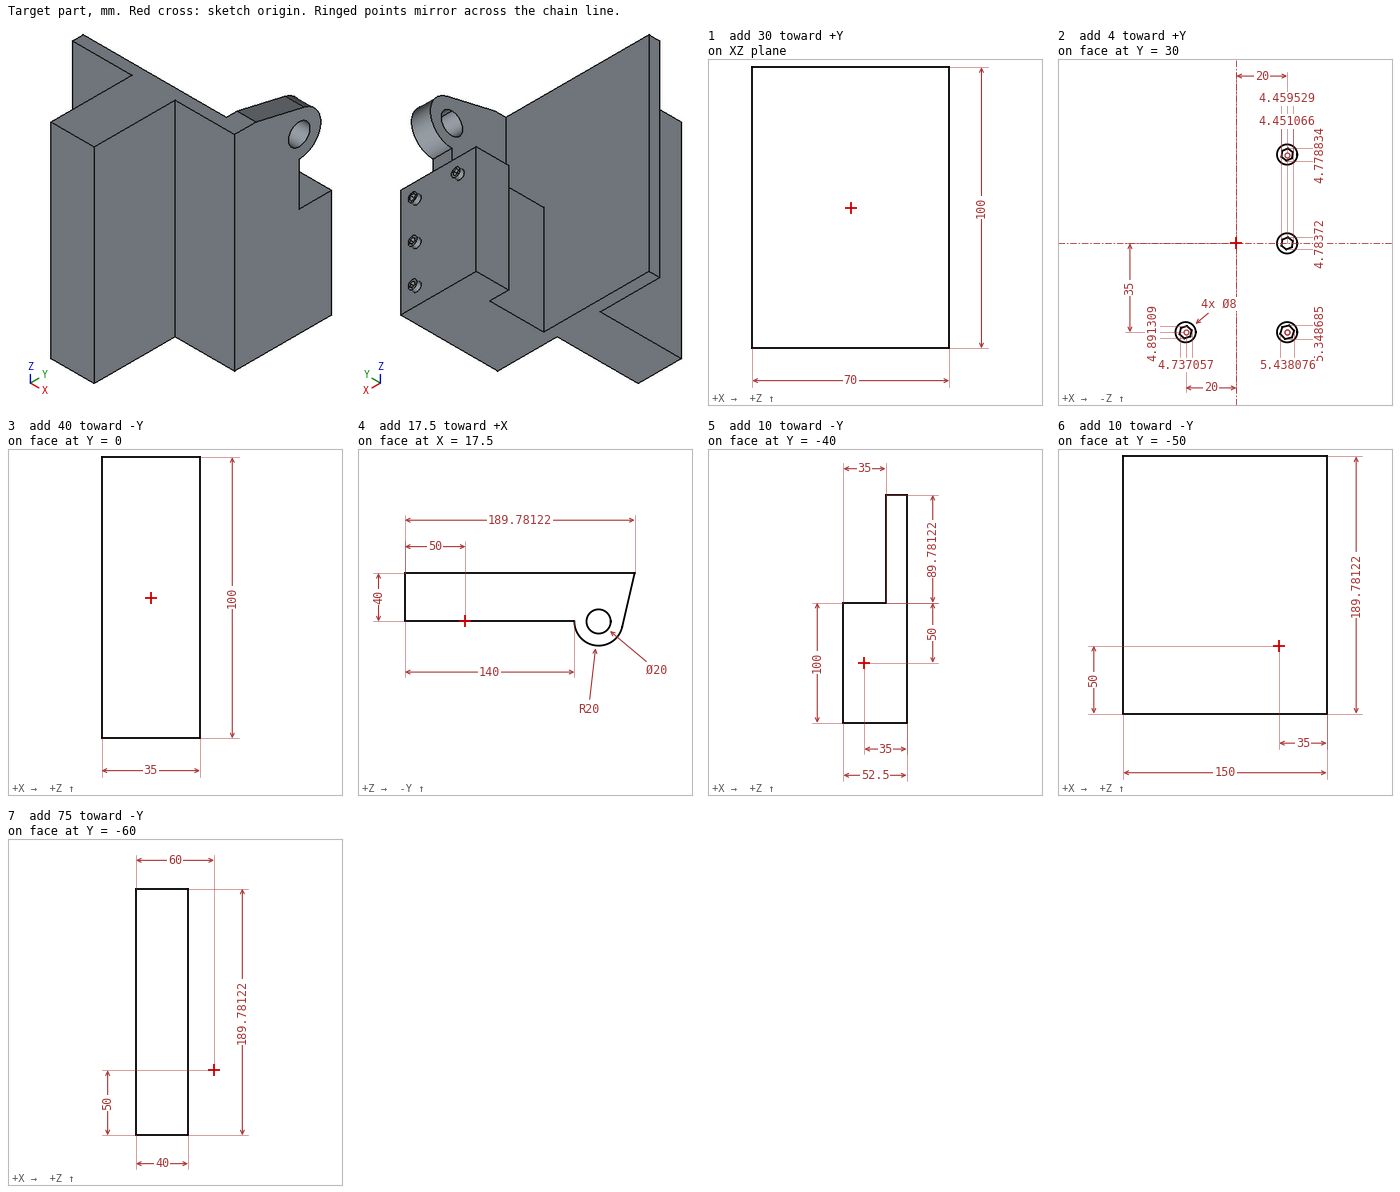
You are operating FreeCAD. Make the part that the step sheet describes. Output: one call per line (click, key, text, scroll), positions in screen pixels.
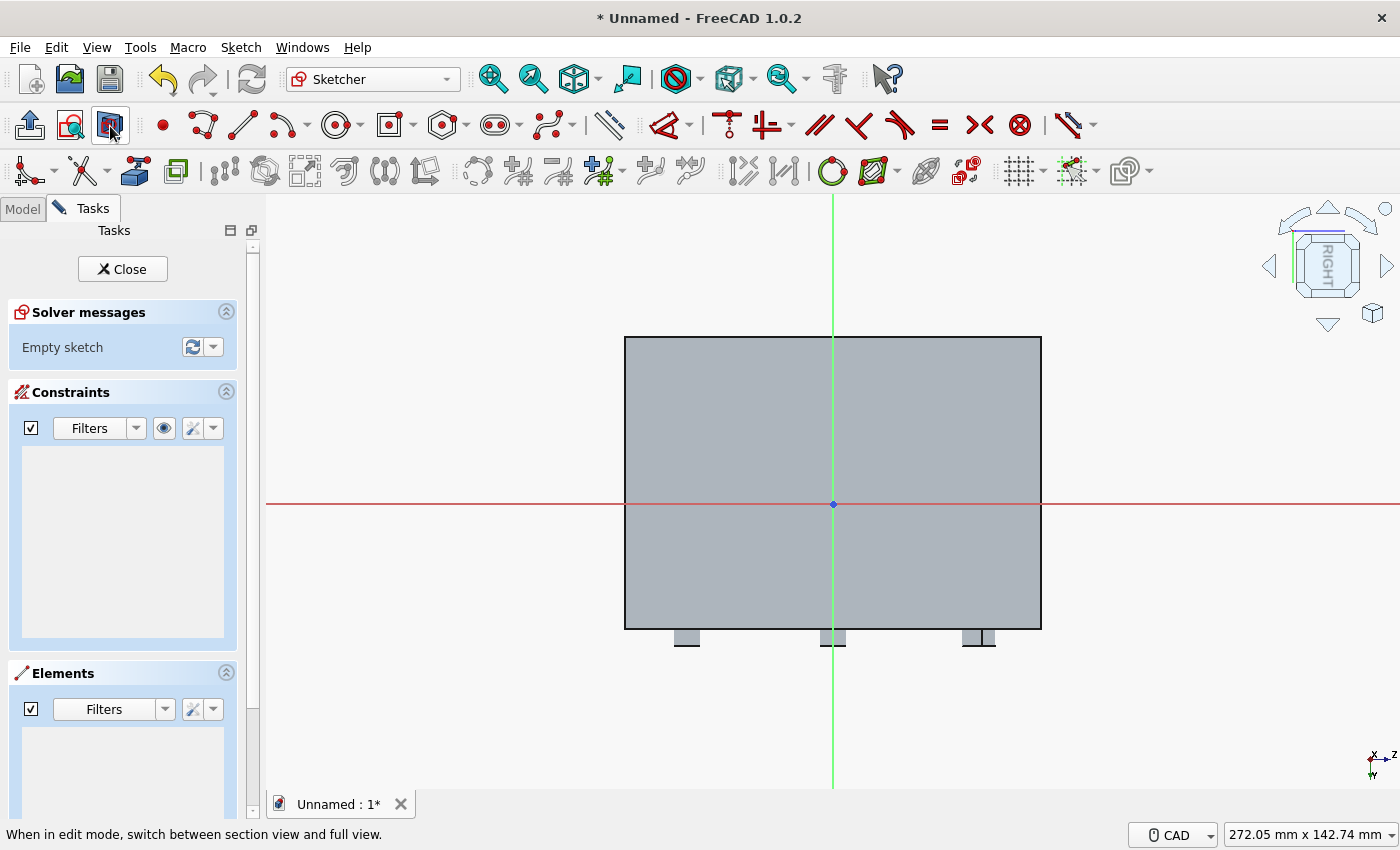
scroll(294, 551, down, 2)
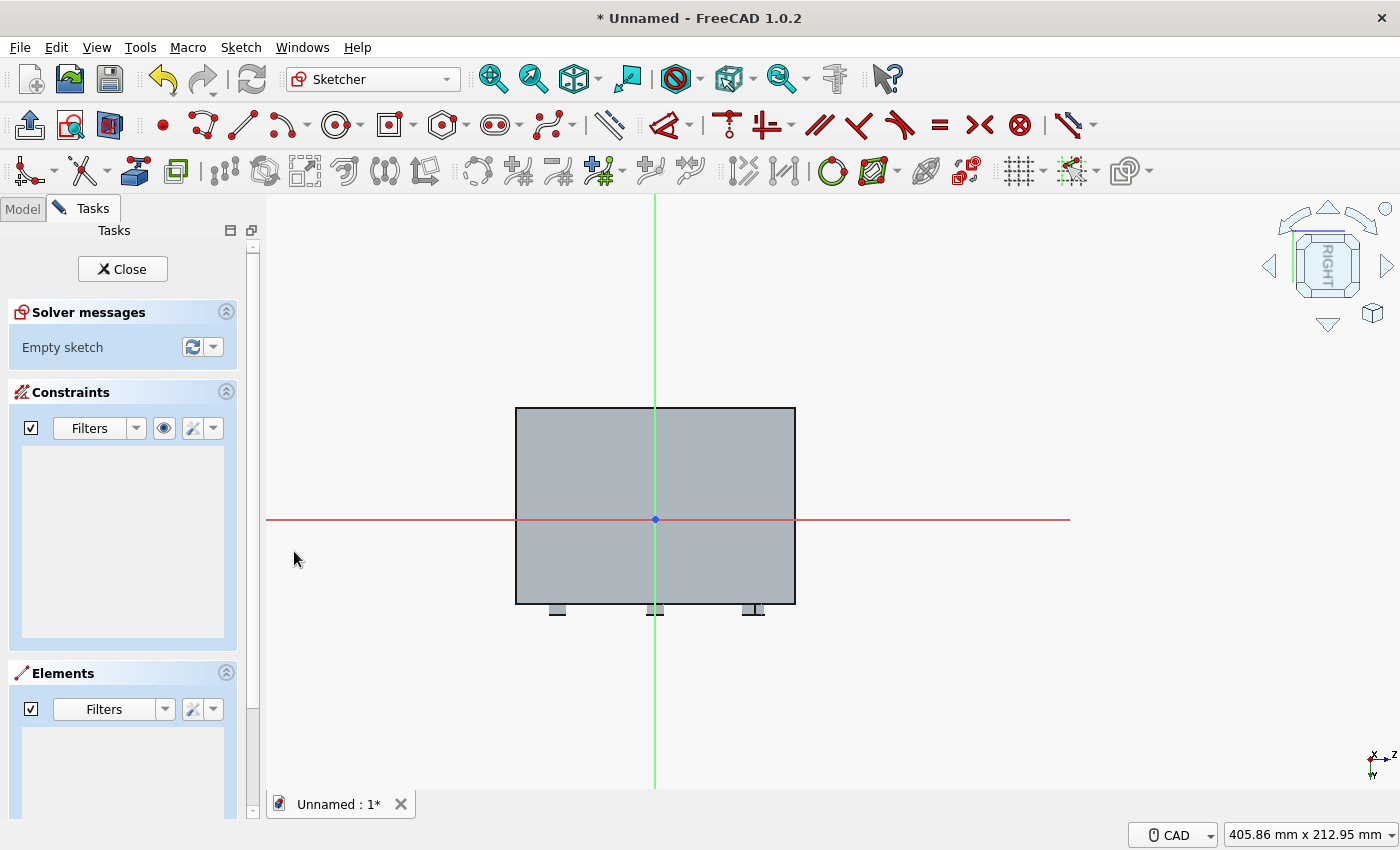
key(g)
key(m)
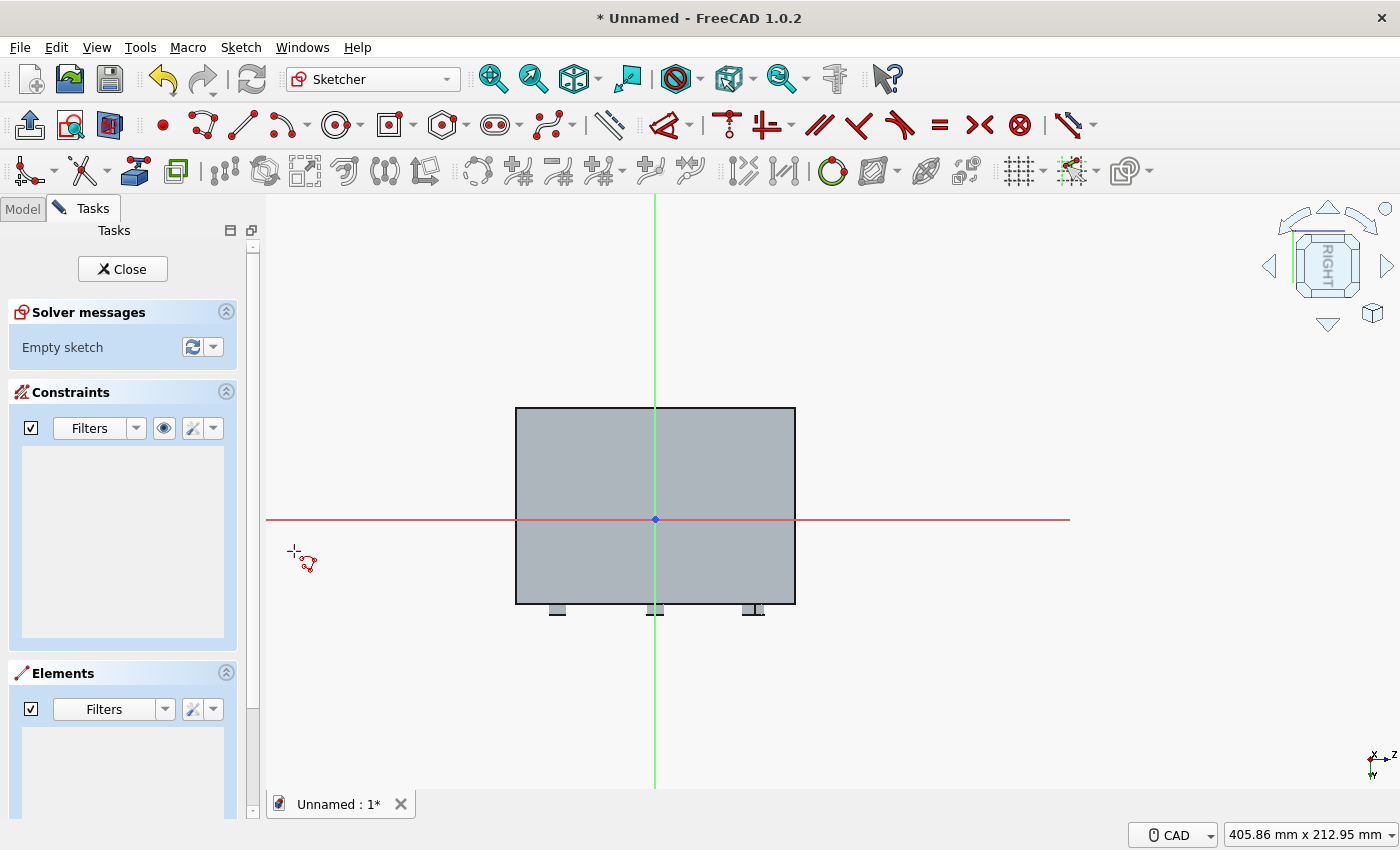
scroll(1017, 532, up, 2)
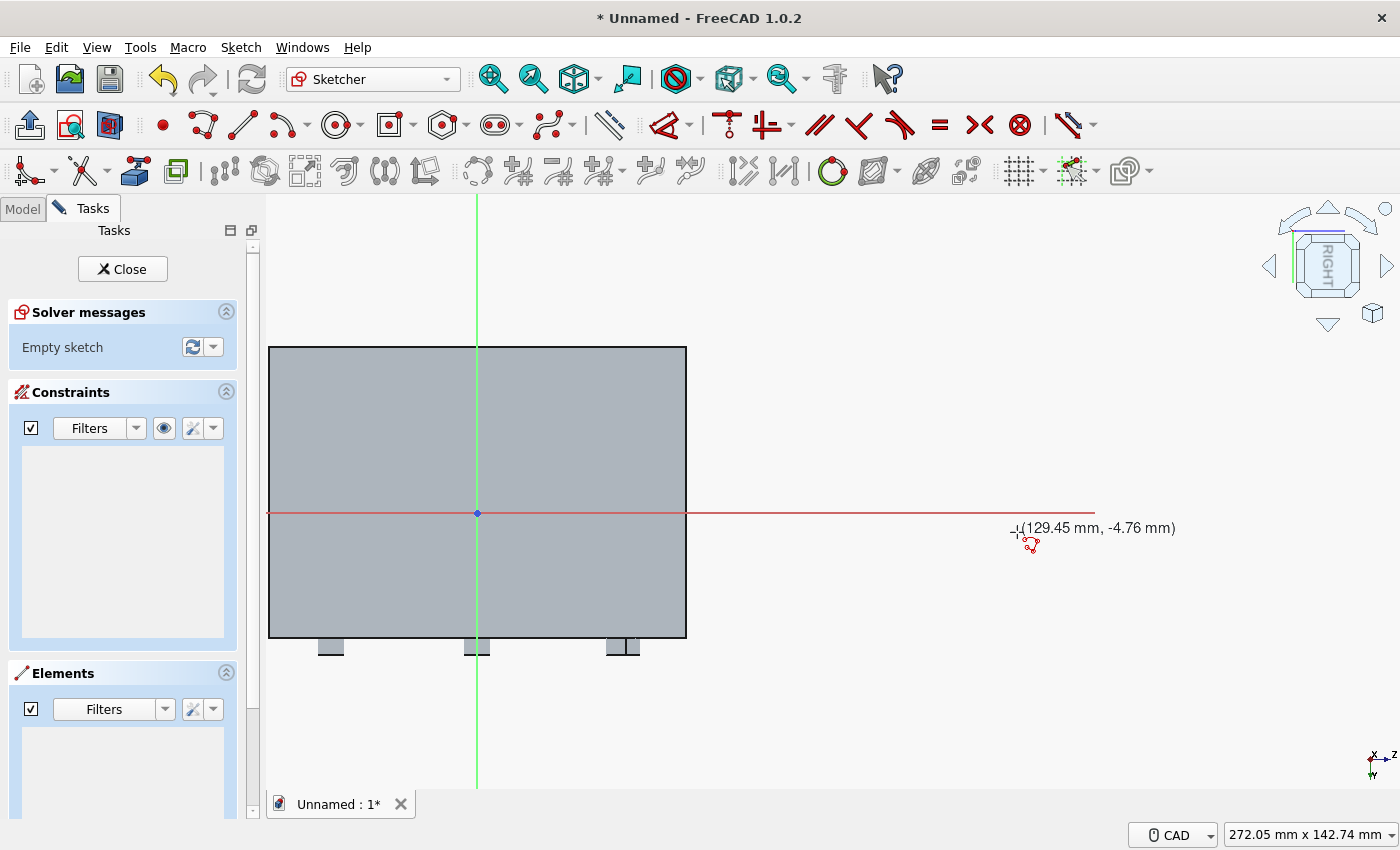
click(1017, 532)
click(1060, 347)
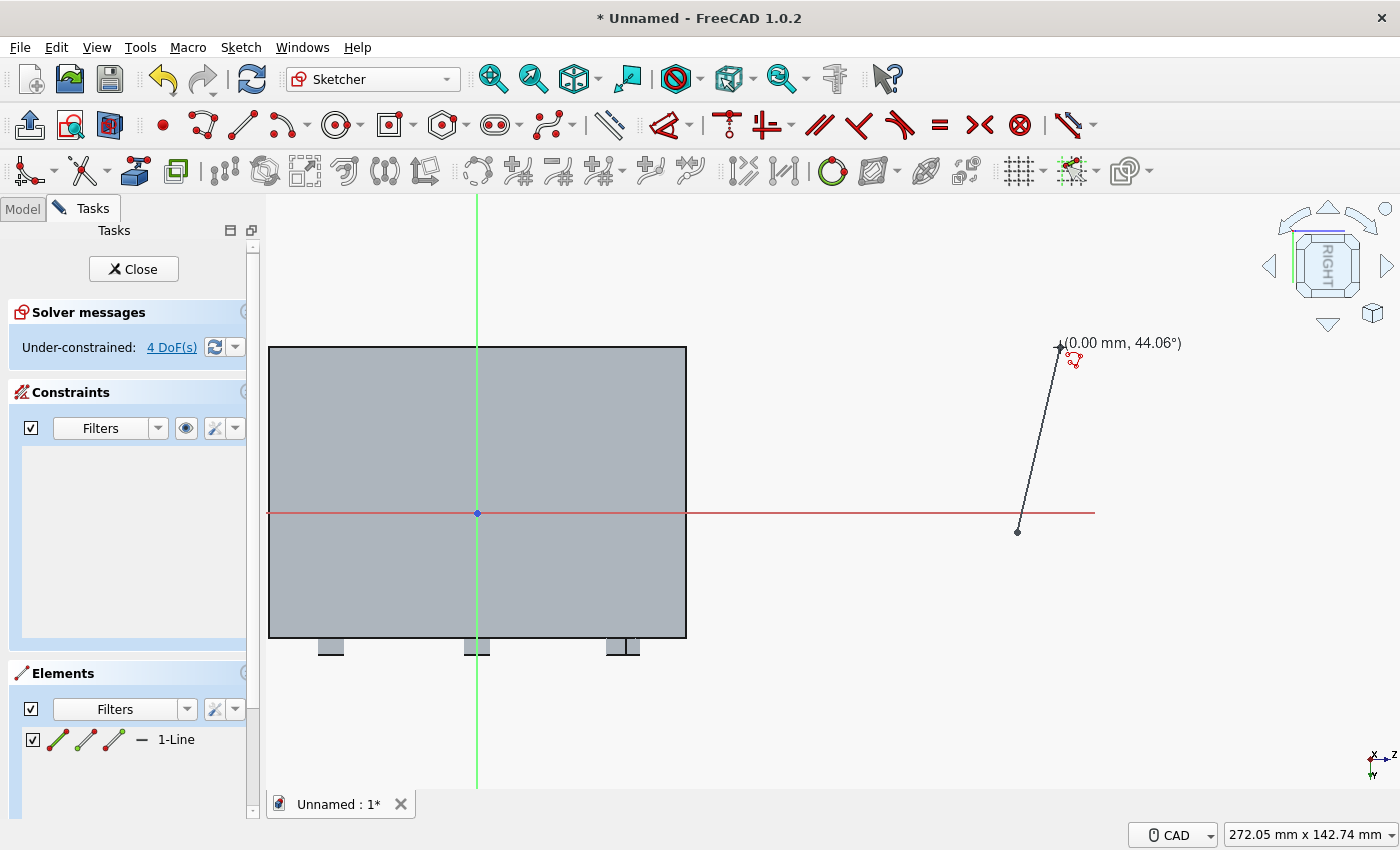
scroll(1217, 582, down, 1)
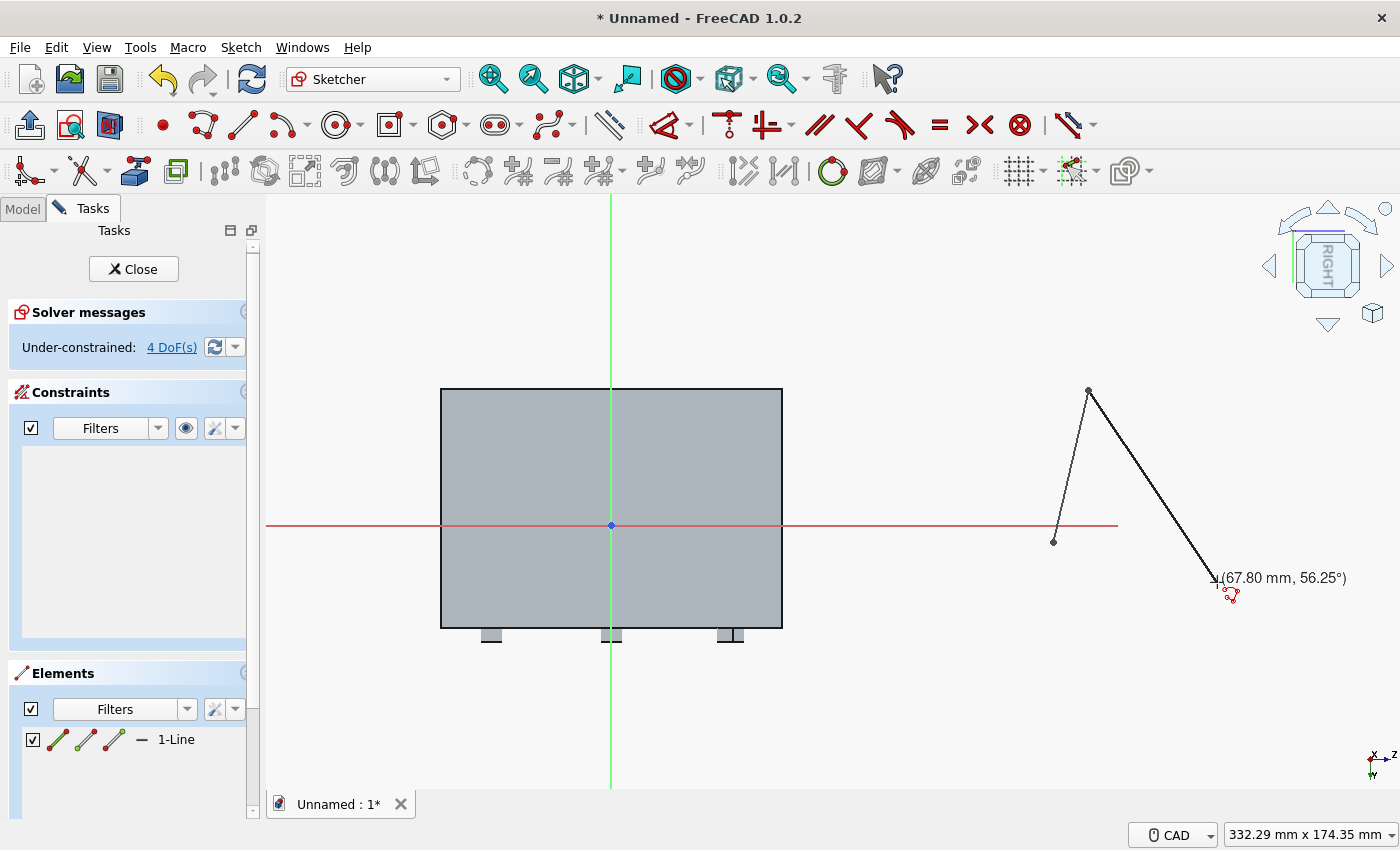
click(441, 390)
click(441, 526)
click(919, 517)
right_click(919, 517)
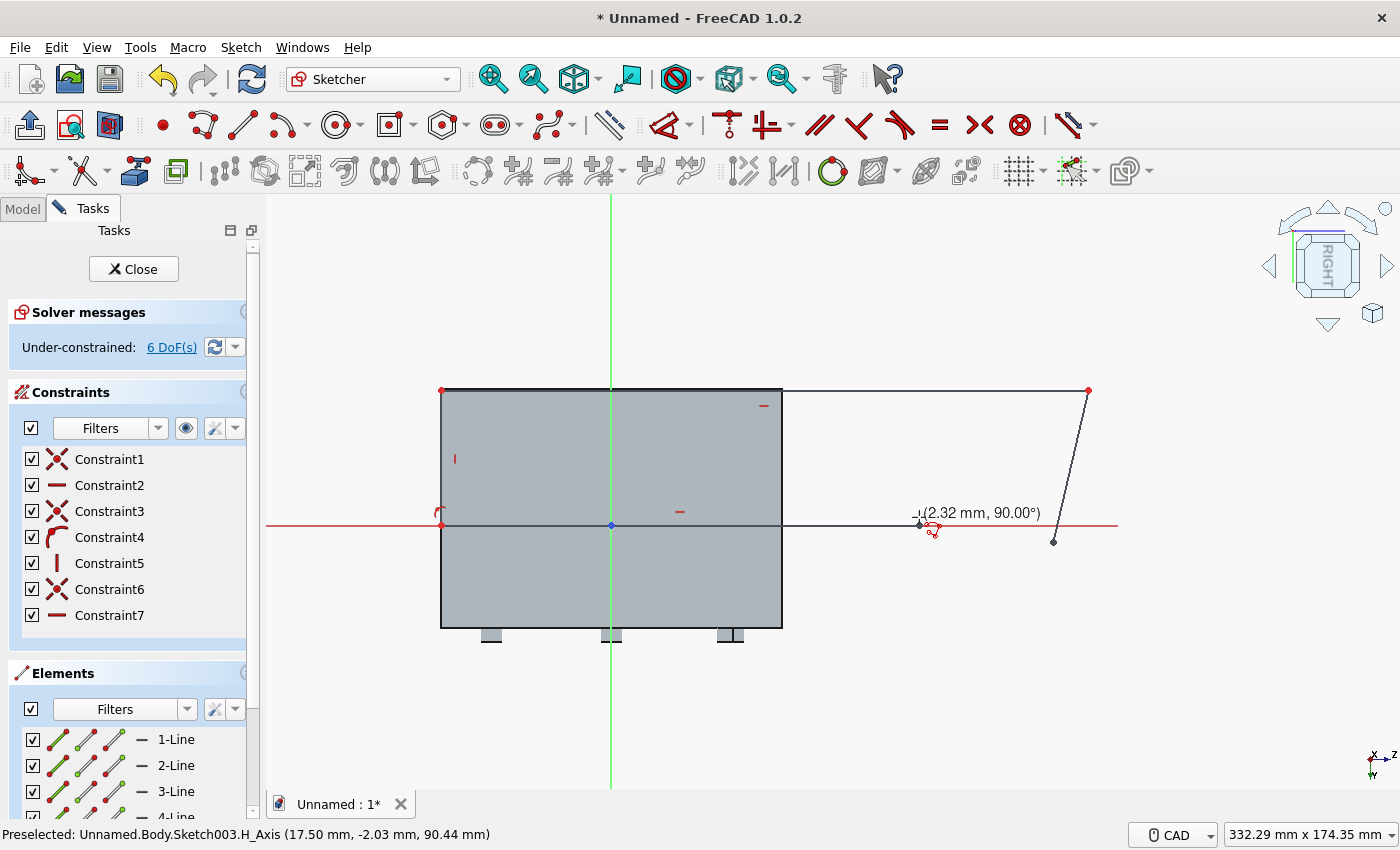
click(310, 126)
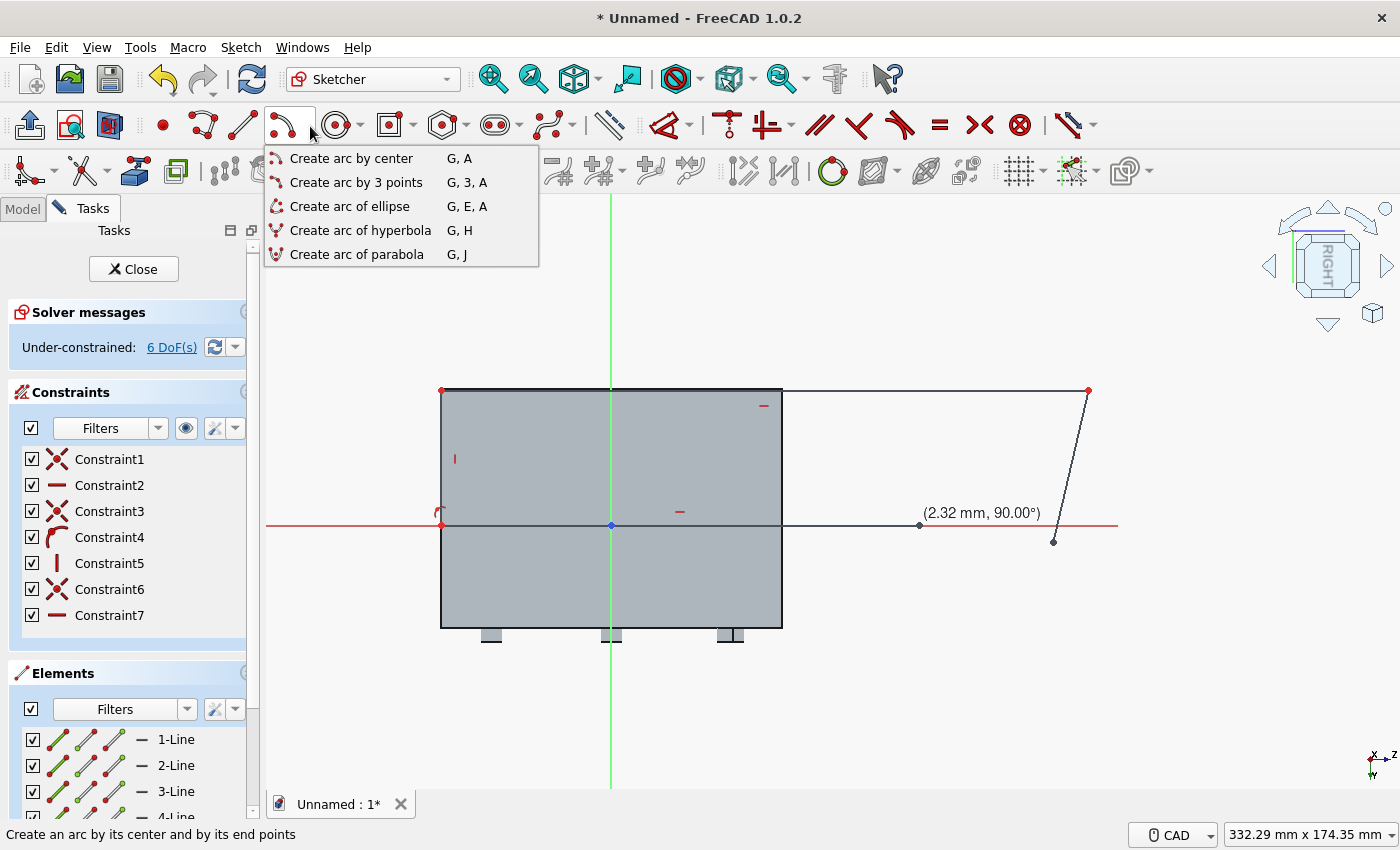
click(402, 182)